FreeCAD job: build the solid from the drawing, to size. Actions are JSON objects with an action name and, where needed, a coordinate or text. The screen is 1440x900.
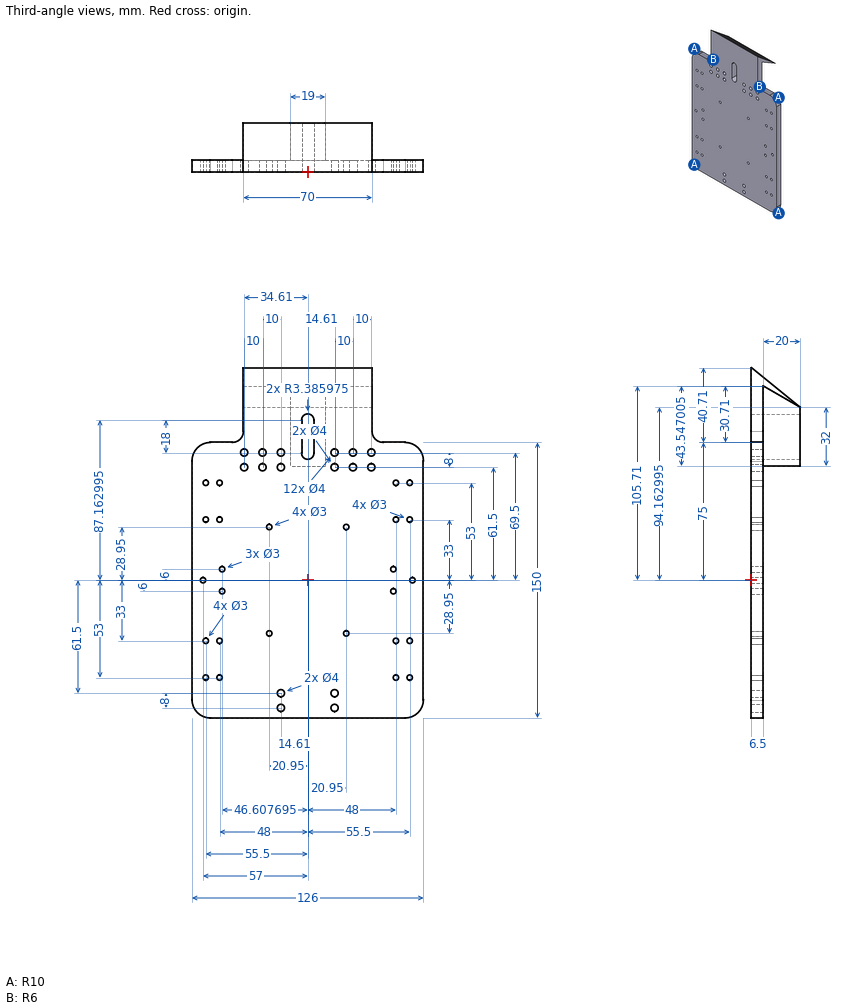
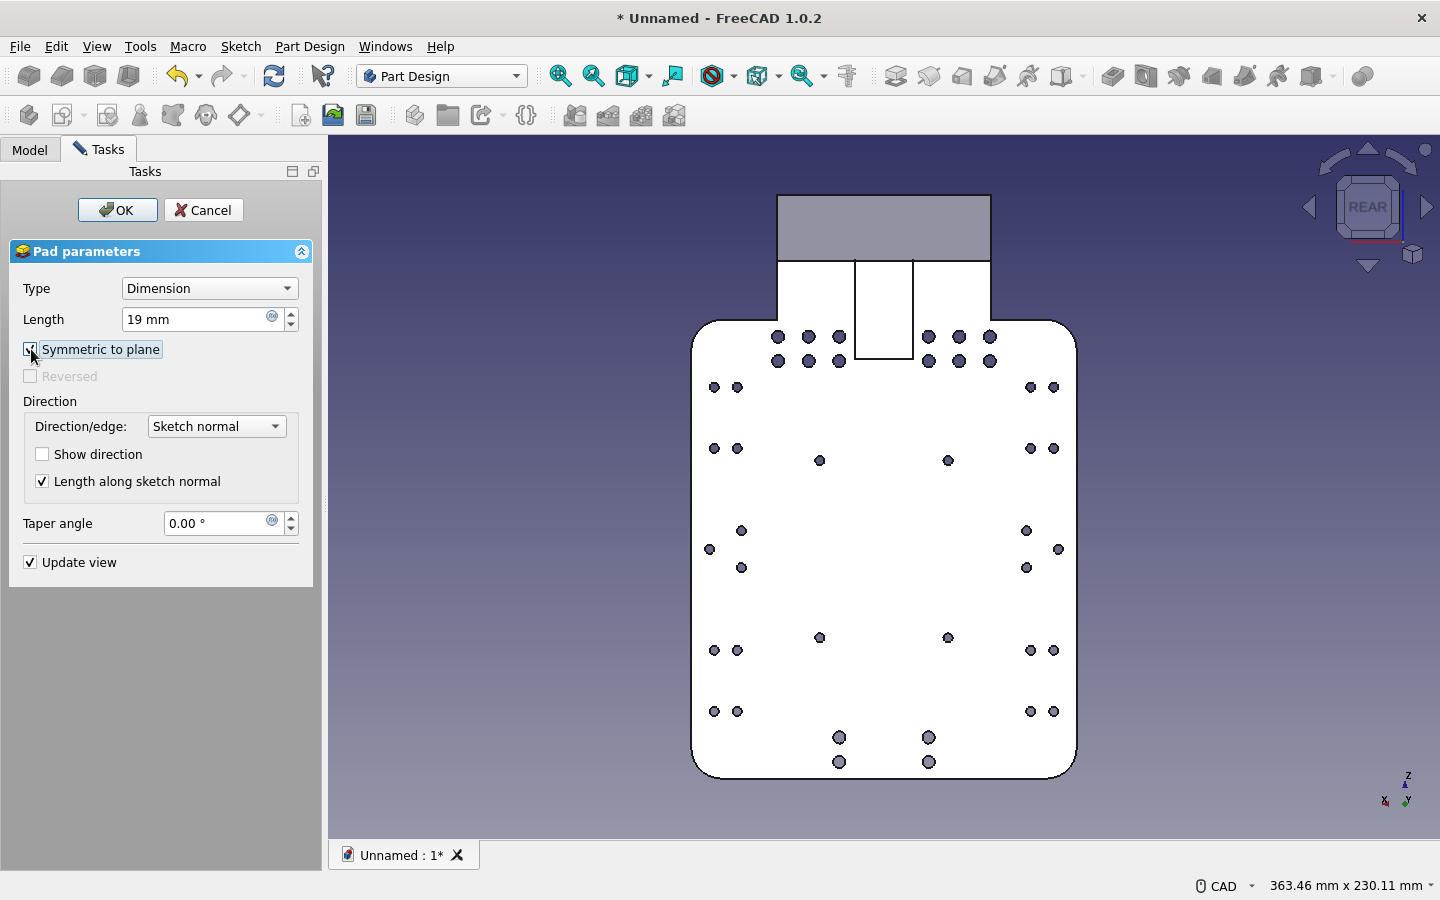
{"action": "left_click", "coordinate": [118, 210]}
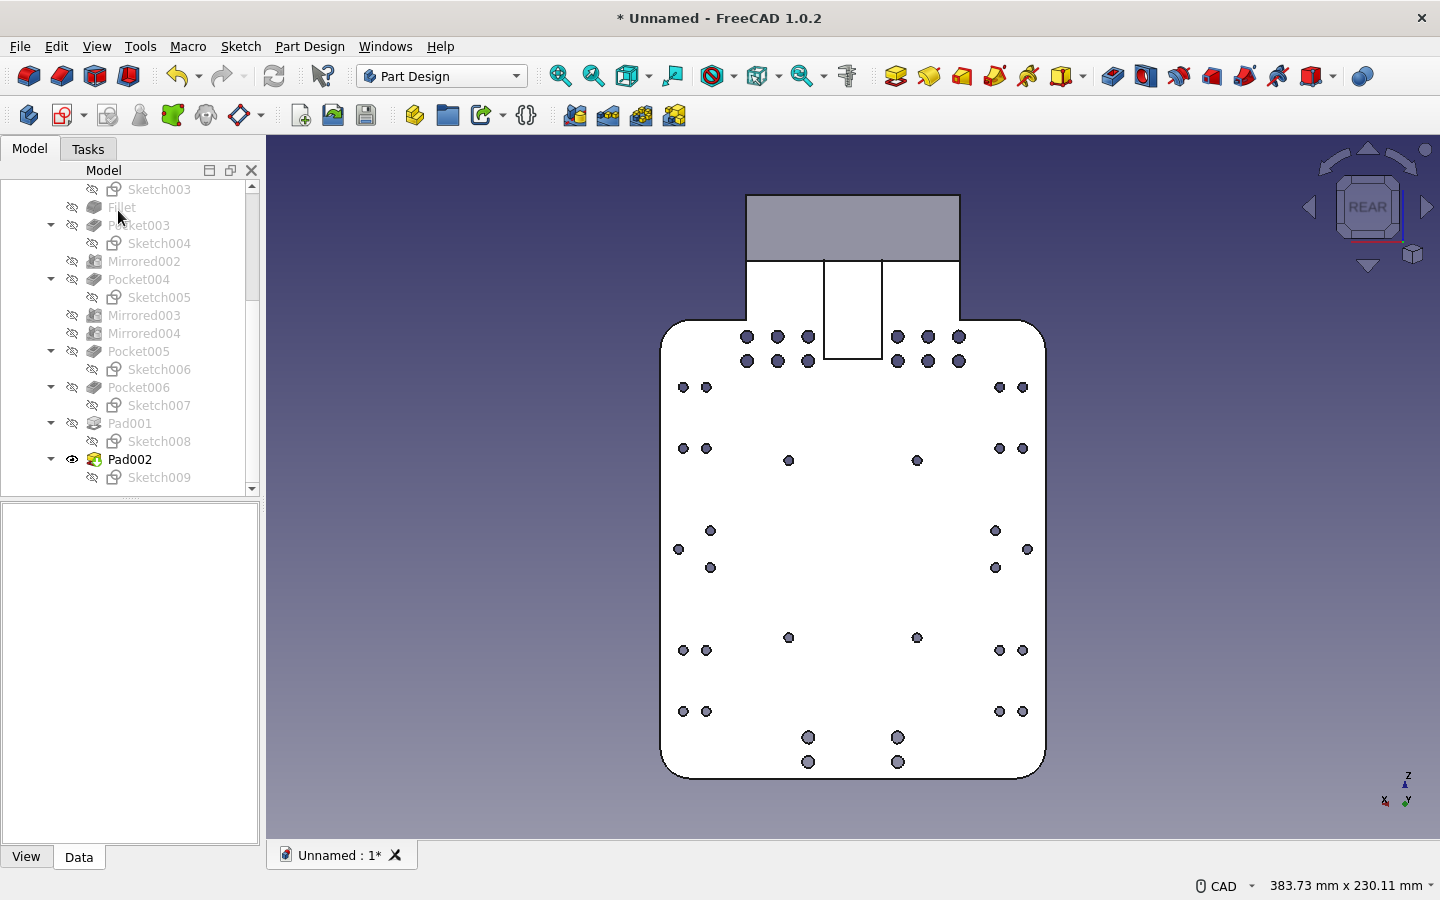
{"action": "left_click", "coordinate": [853, 295]}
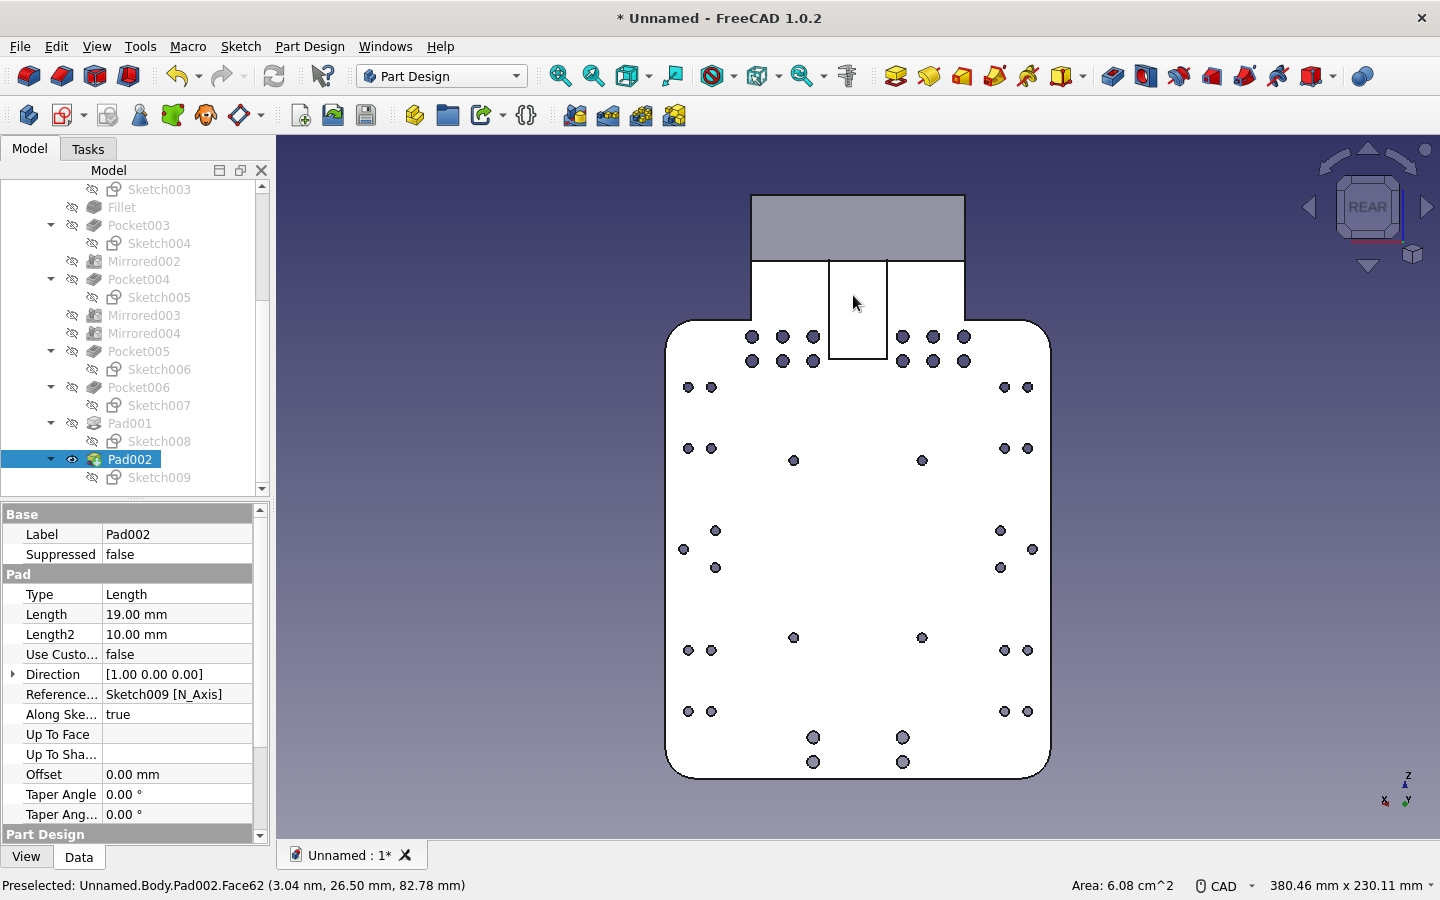
{"action": "left_click", "coordinate": [62, 116]}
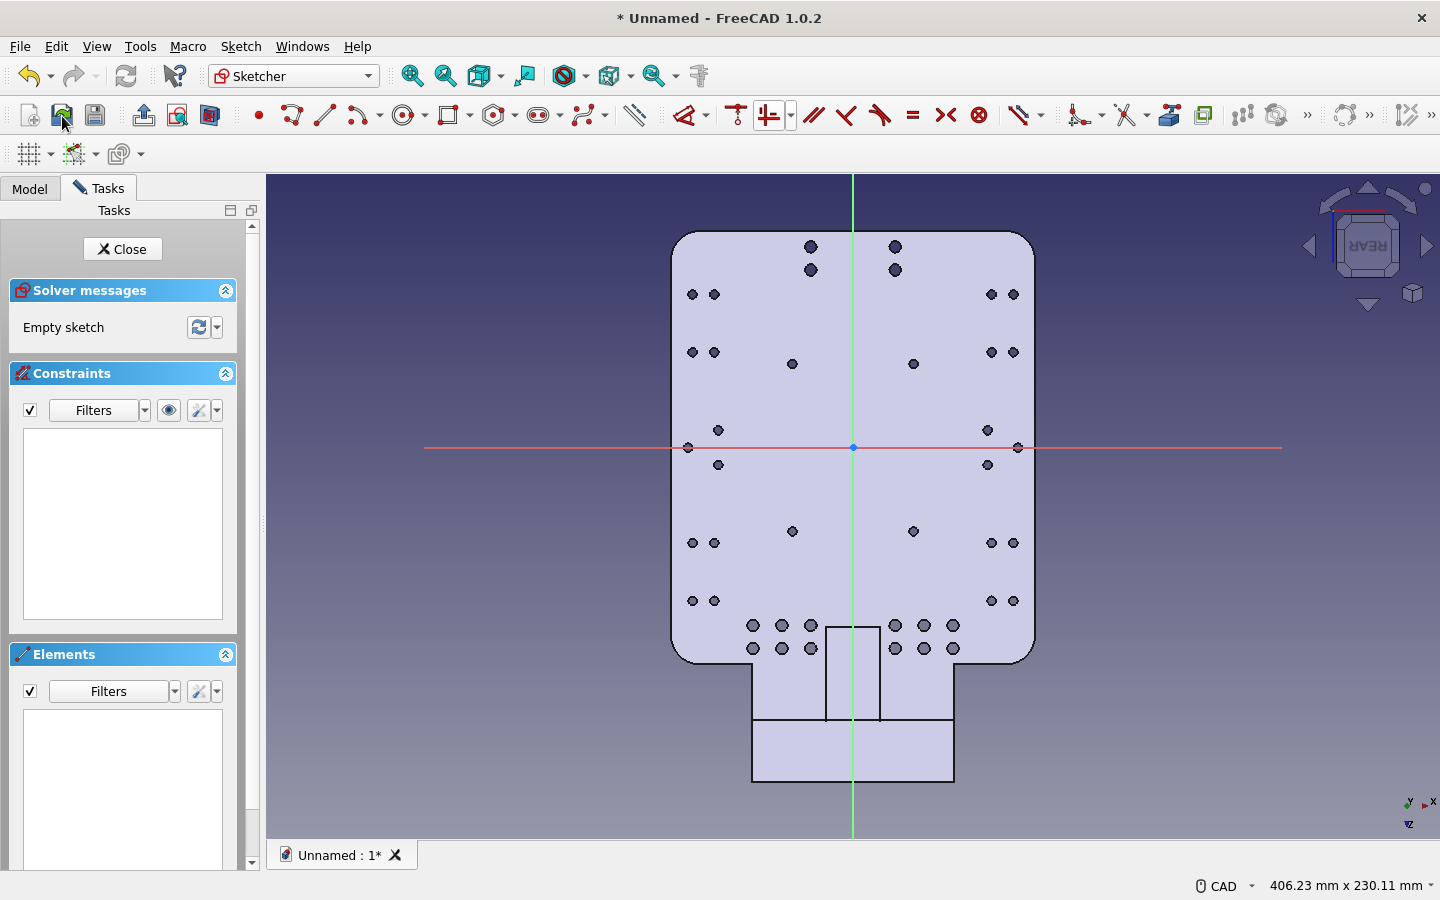
{"action": "scroll", "coordinate": [867, 707], "scroll_direction": "up", "scroll_amount": 9}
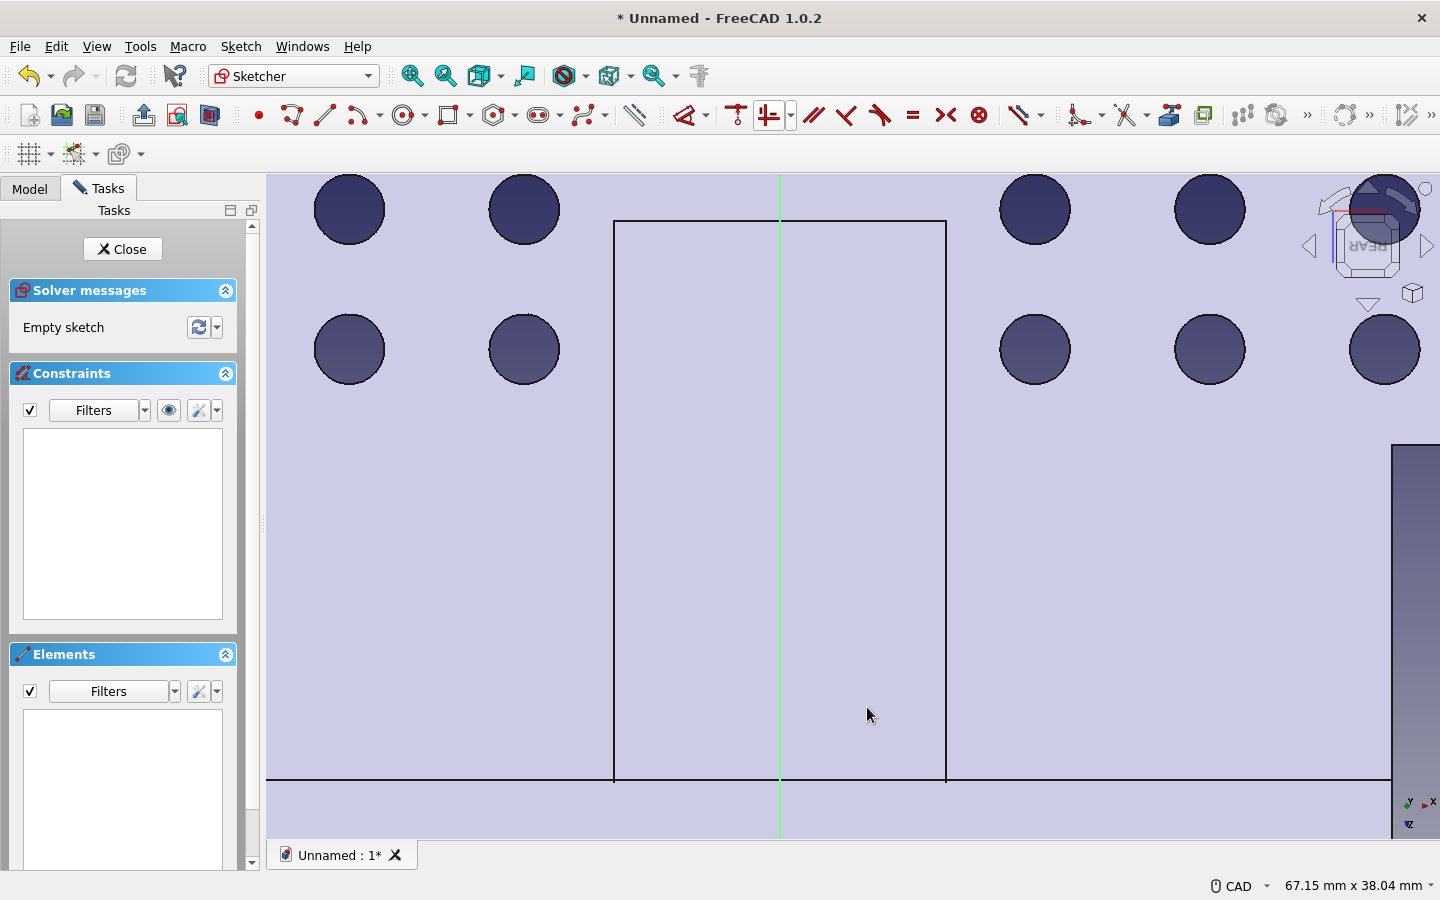
{"action": "left_click", "coordinate": [538, 116]}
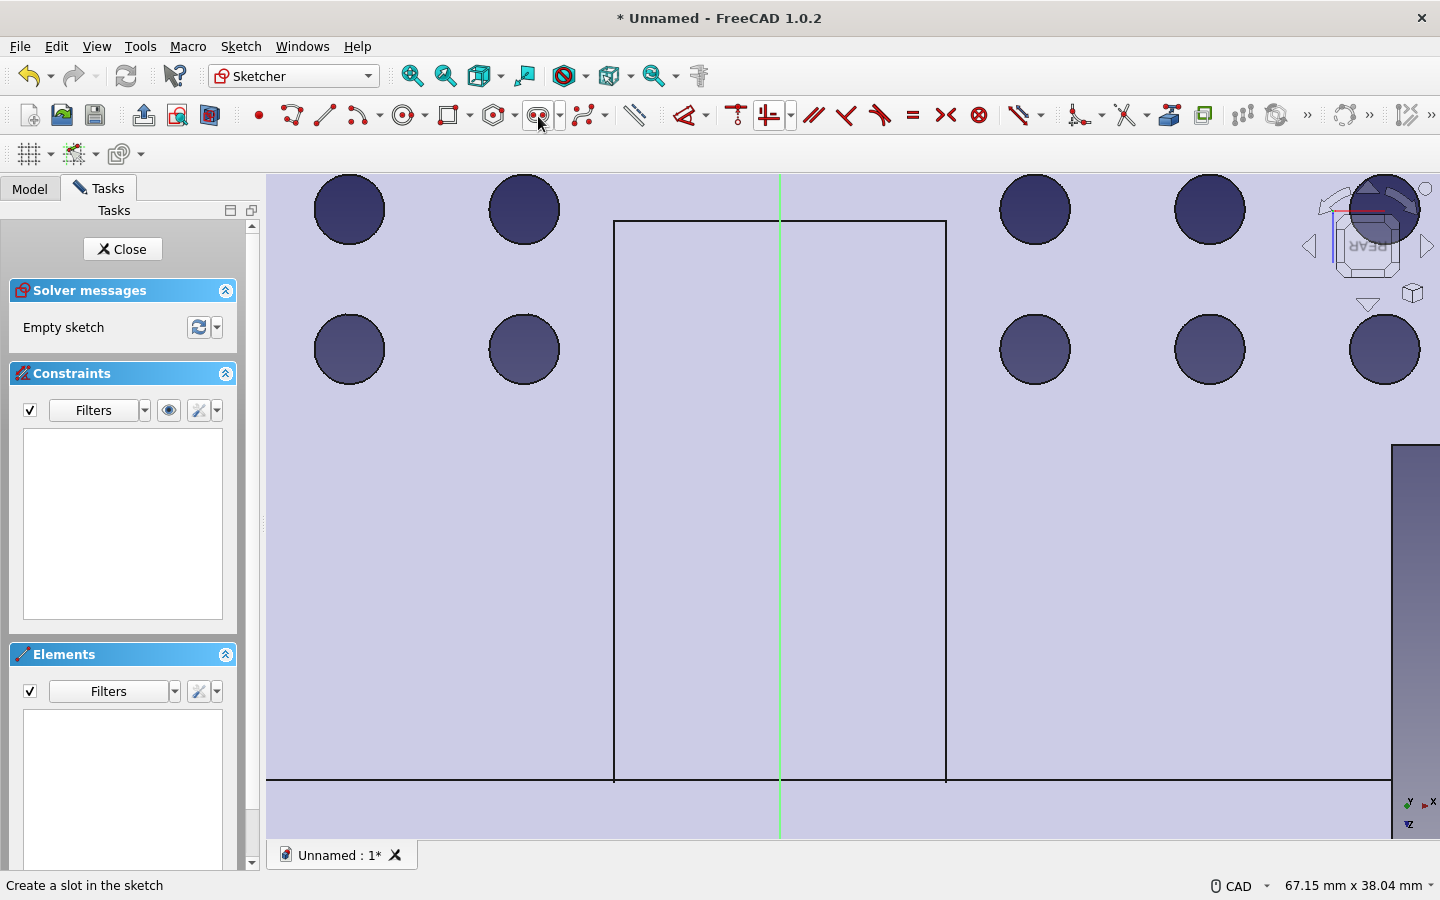
{"action": "left_click", "coordinate": [780, 658]}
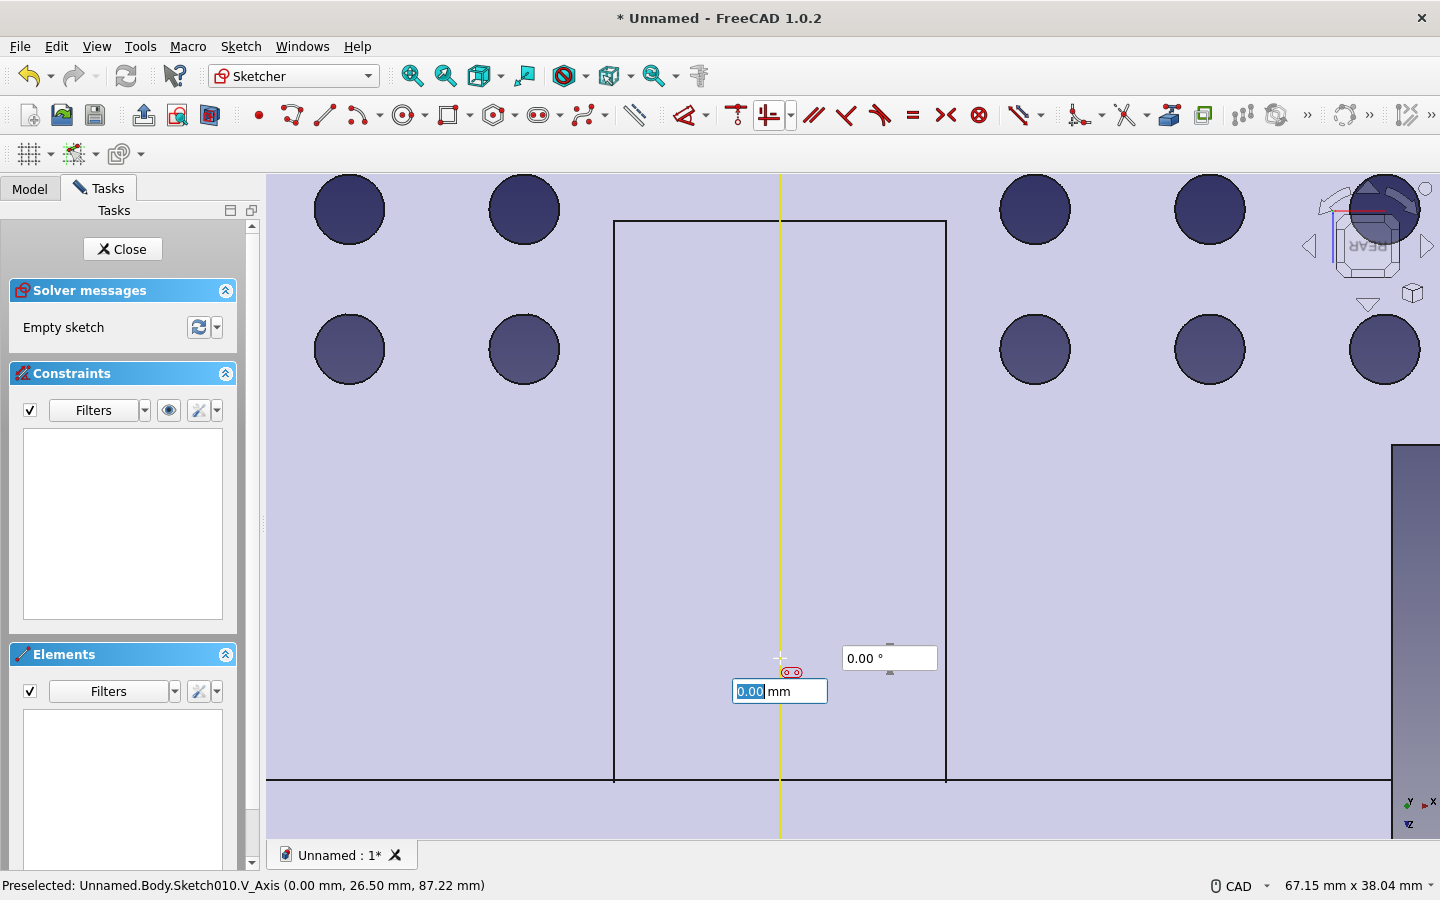
{"action": "left_click", "coordinate": [789, 343]}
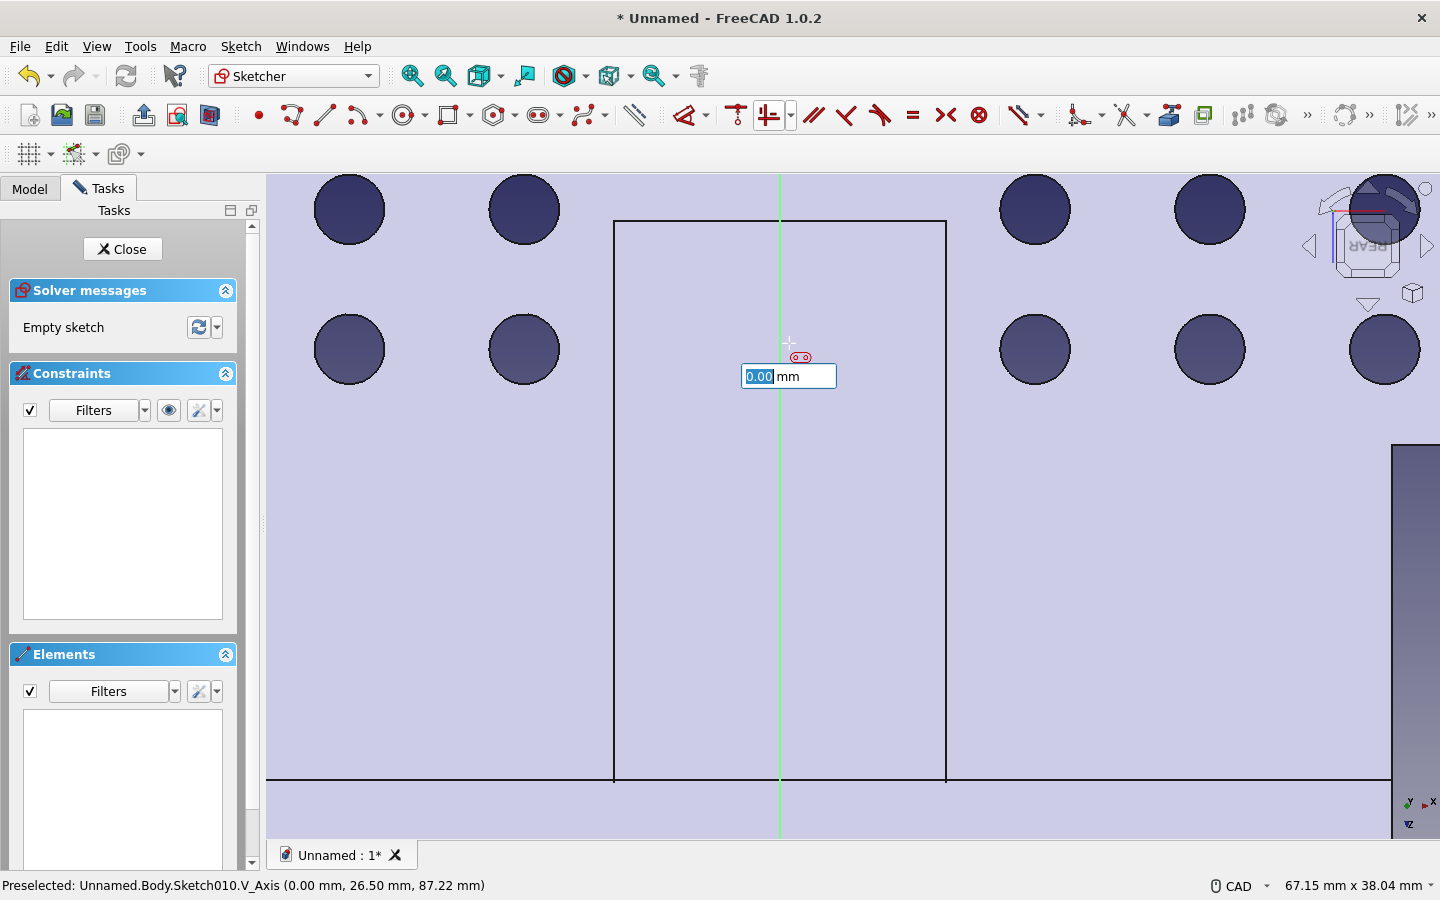
{"action": "left_click", "coordinate": [721, 501]}
{"action": "key", "text": "Escape"}